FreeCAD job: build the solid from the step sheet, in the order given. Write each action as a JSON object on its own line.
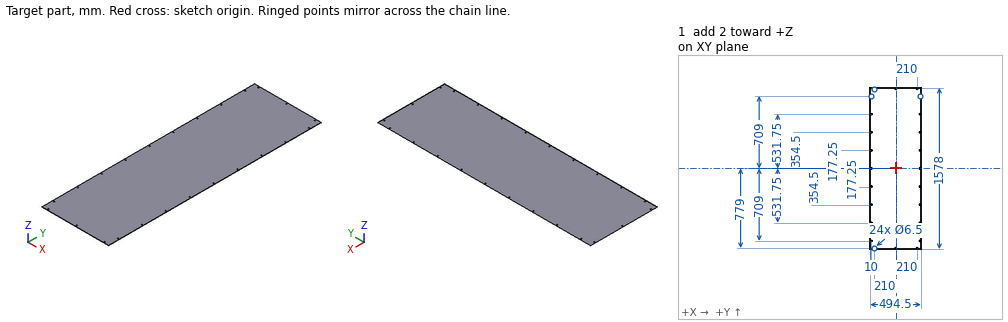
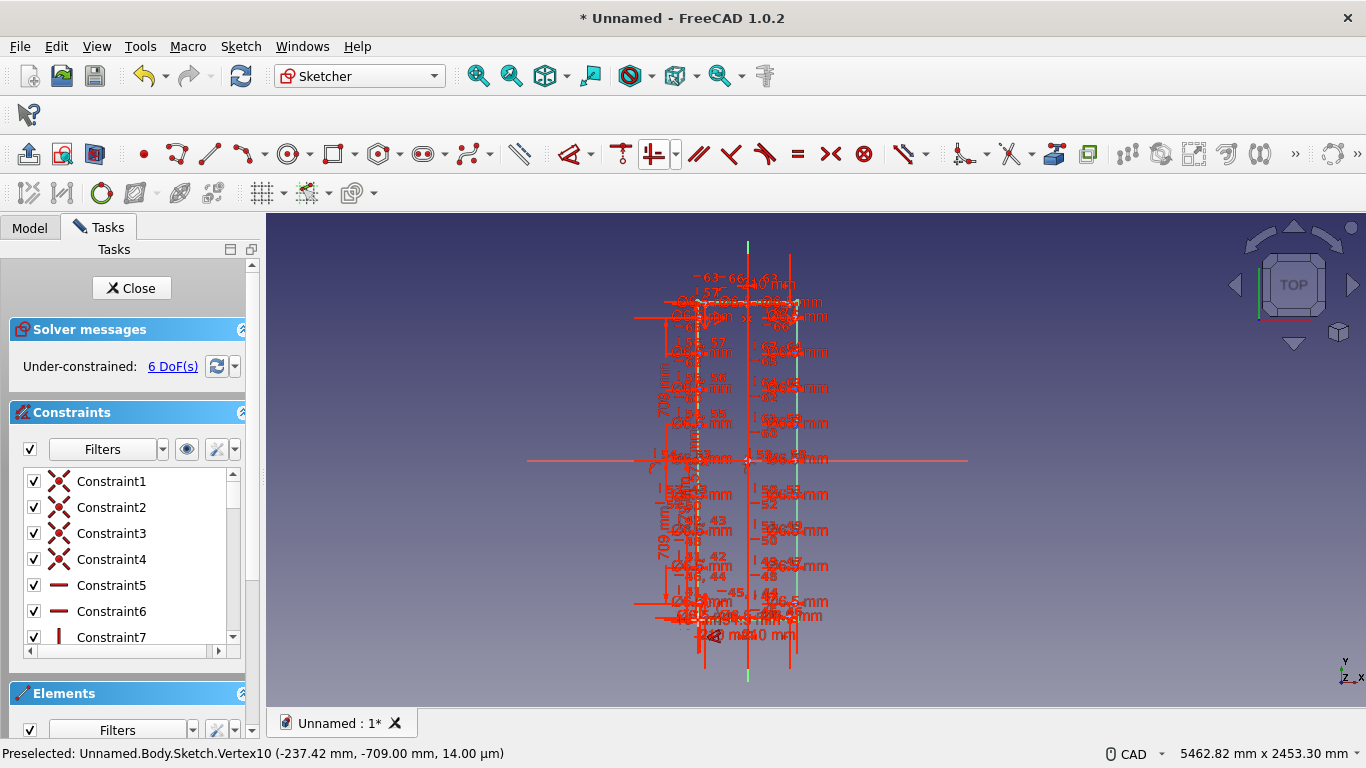
{"action": "left_click", "coordinate": [700, 532]}
{"action": "left_click", "coordinate": [666, 480]}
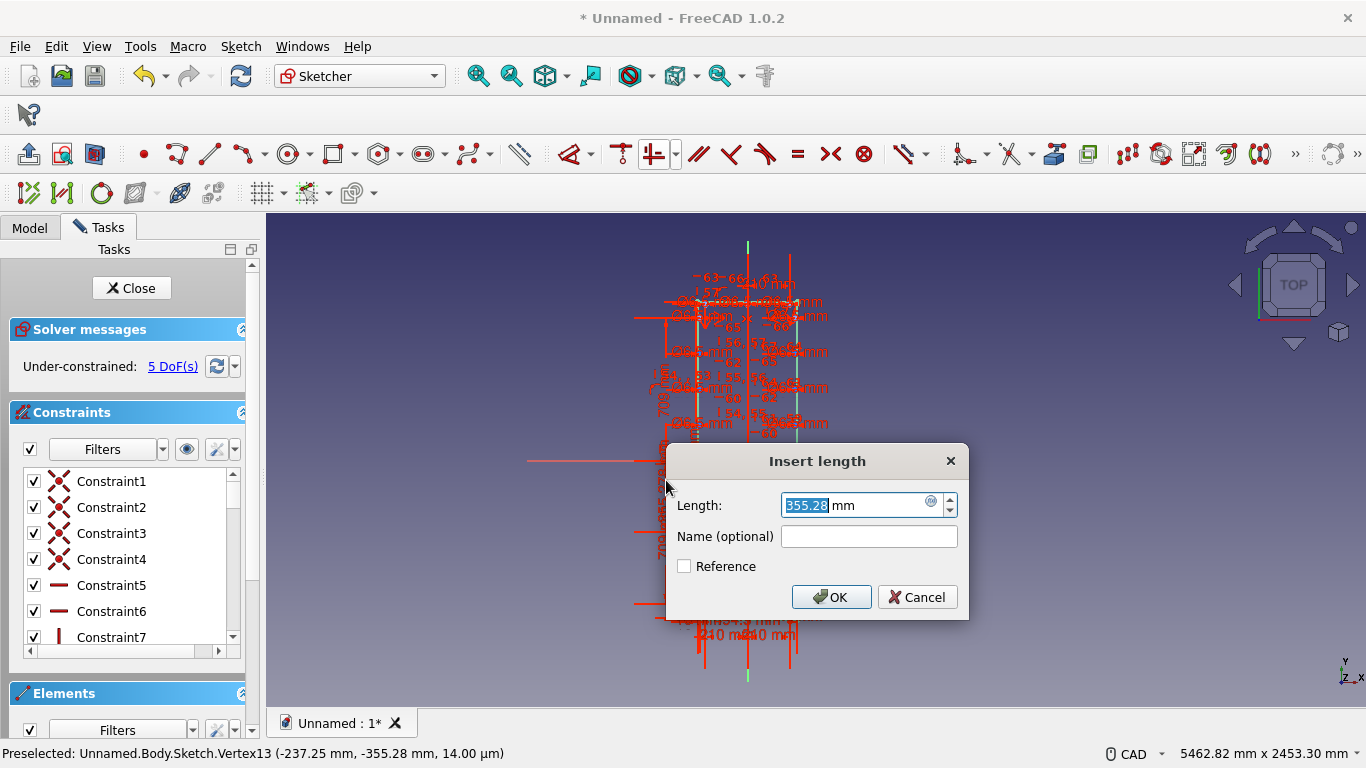
{"action": "type", "text": "354.5"}
{"action": "key", "text": "Return"}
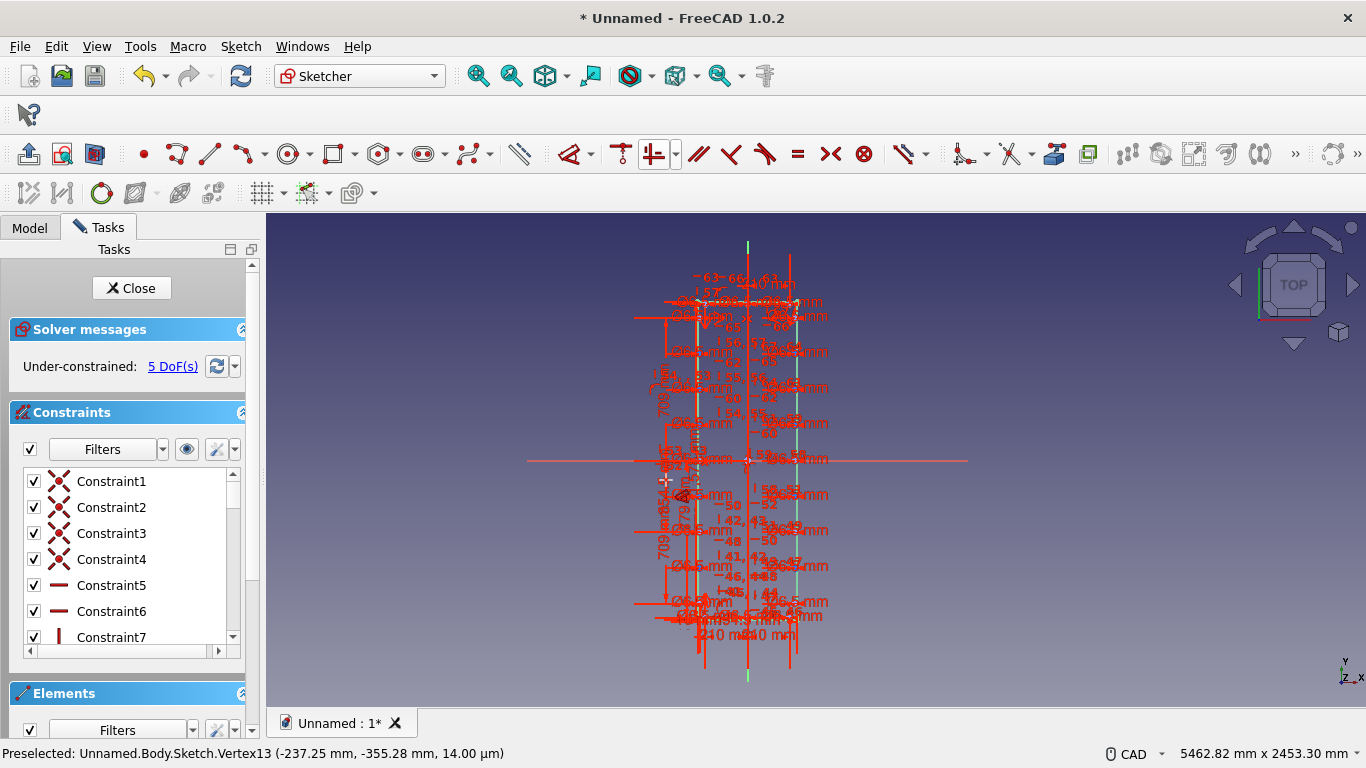
{"action": "left_click", "coordinate": [700, 390]}
{"action": "left_click", "coordinate": [666, 425]}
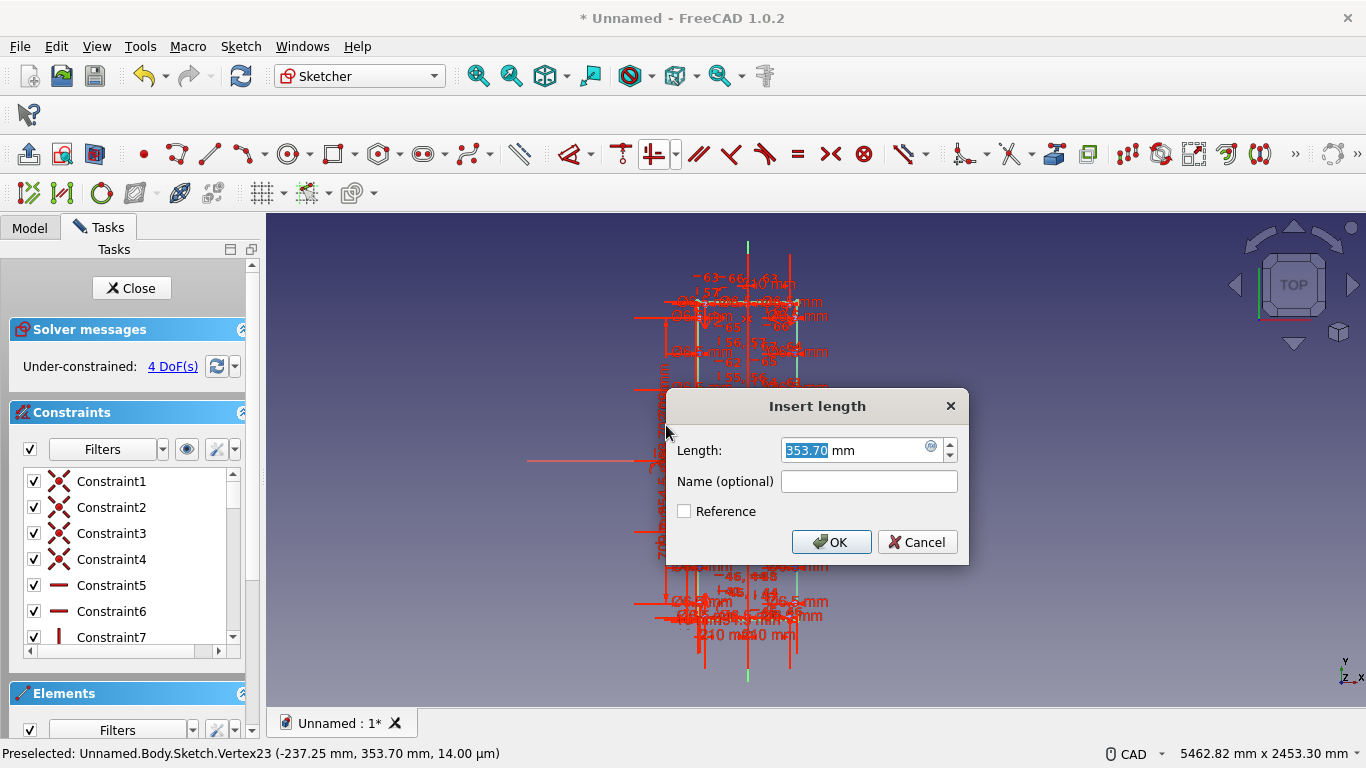
{"action": "type", "text": "354.5"}
{"action": "key", "text": "Return"}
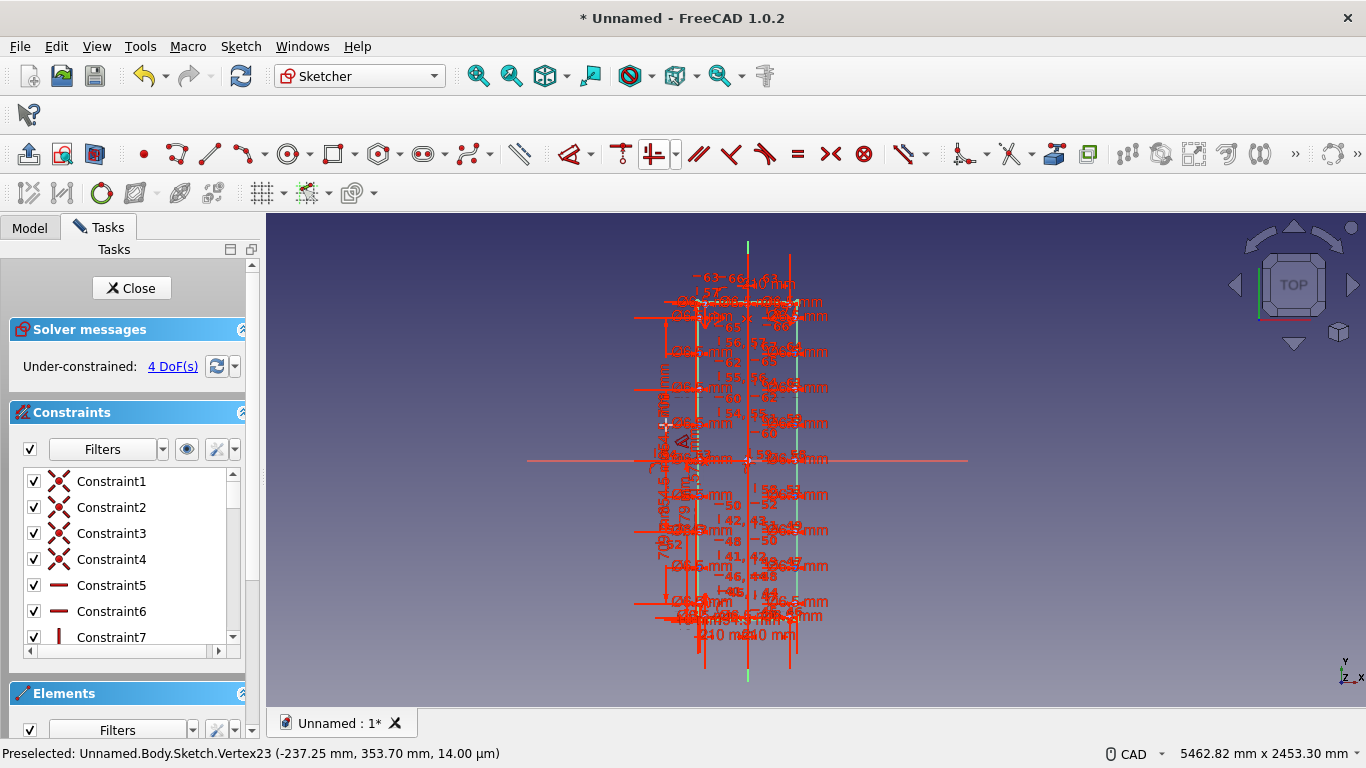
{"action": "left_click", "coordinate": [700, 568]}
{"action": "left_click", "coordinate": [782, 515]}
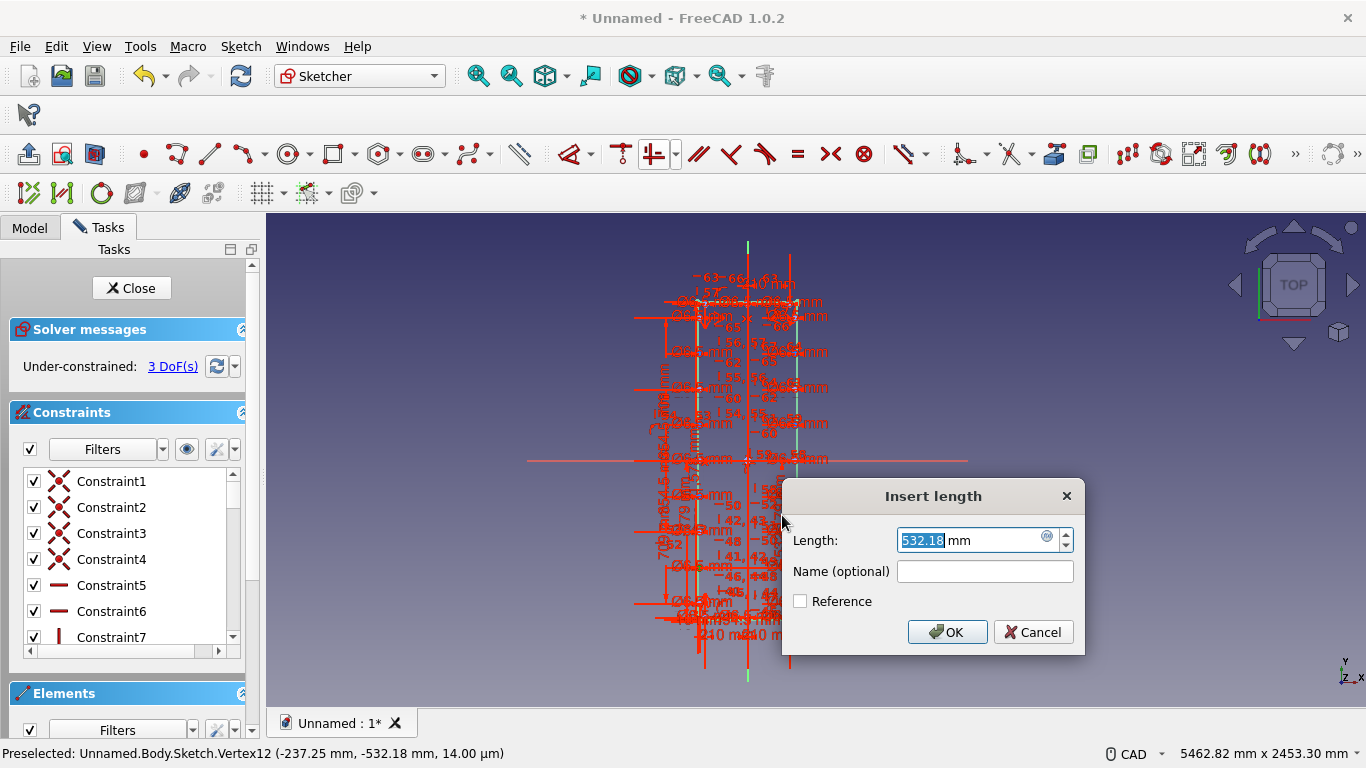
{"action": "type", "text": "531.75"}
{"action": "key", "text": "Return"}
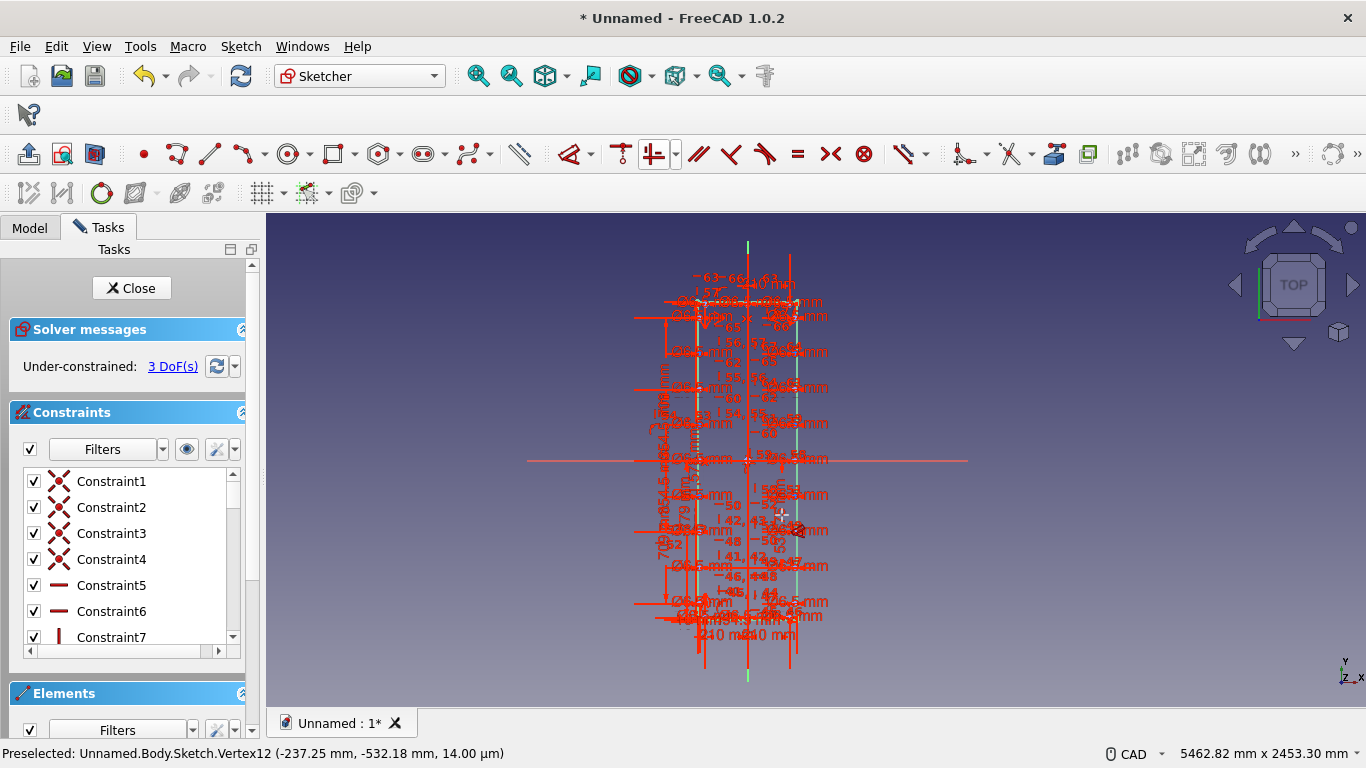
{"action": "left_click", "coordinate": [700, 497]}
{"action": "left_click", "coordinate": [782, 479]}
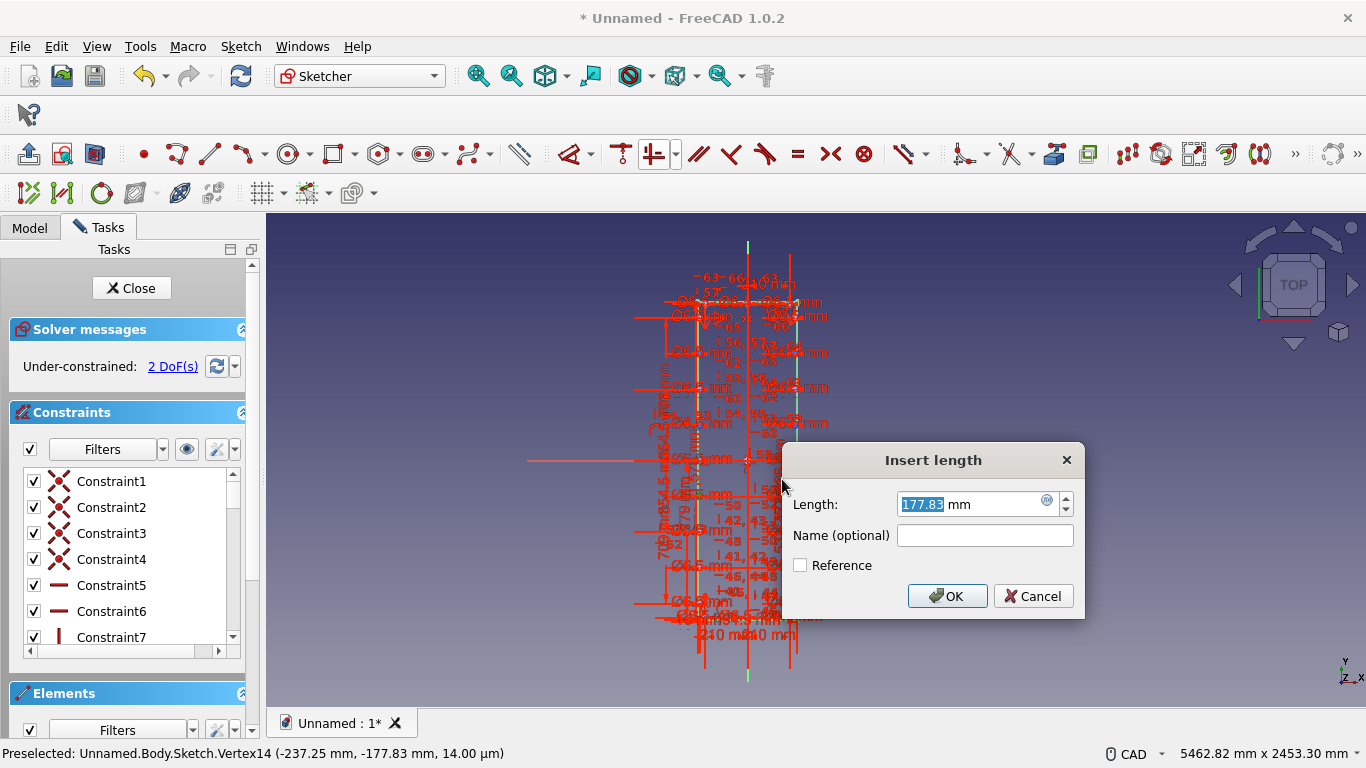
{"action": "type", "text": "177.25"}
{"action": "key", "text": "Return"}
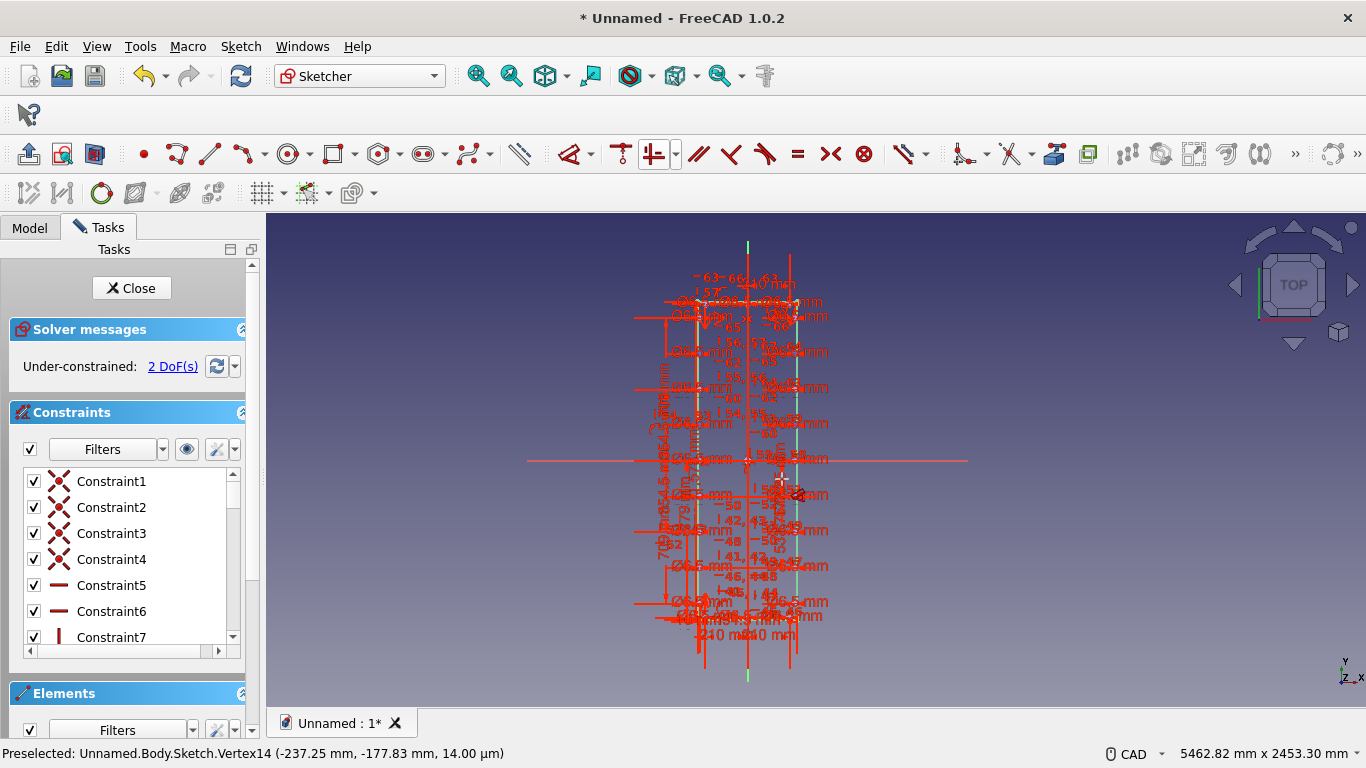
{"action": "left_click", "coordinate": [700, 425]}
{"action": "left_click", "coordinate": [782, 443]}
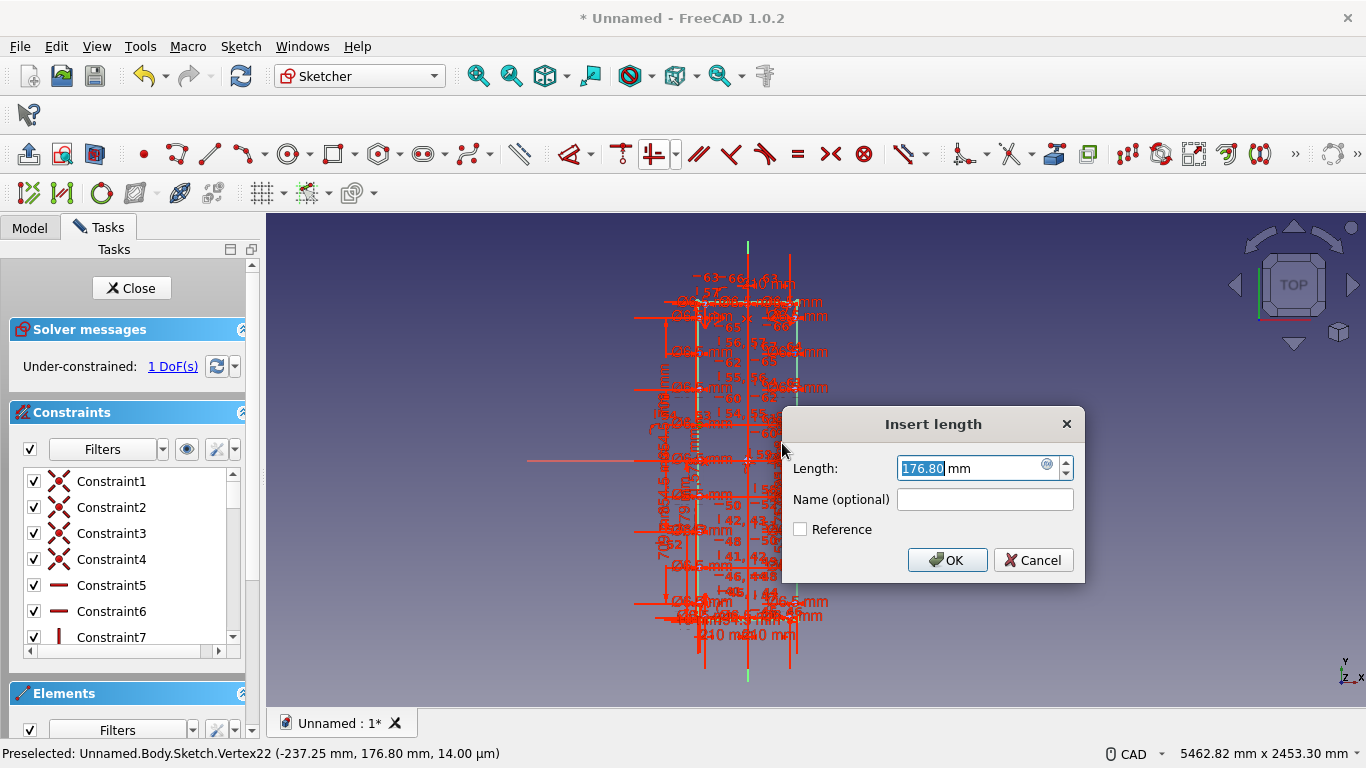
{"action": "type", "text": "177.25"}
{"action": "key", "text": "Return"}